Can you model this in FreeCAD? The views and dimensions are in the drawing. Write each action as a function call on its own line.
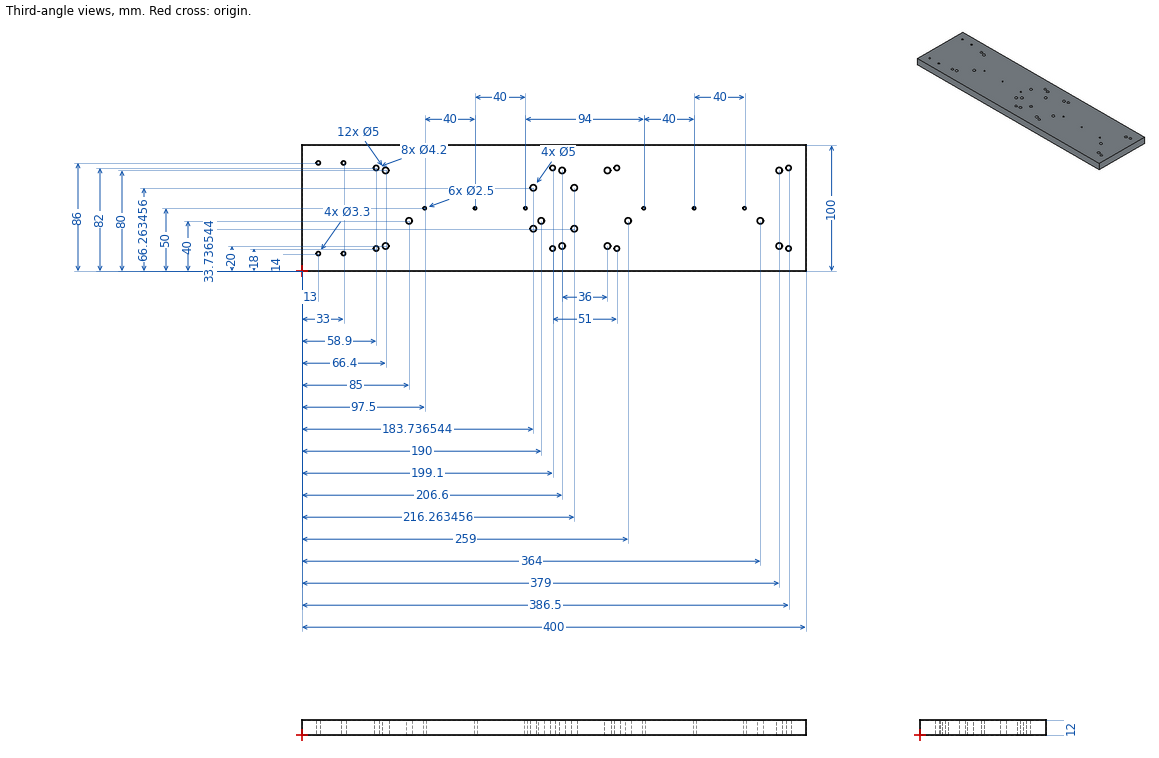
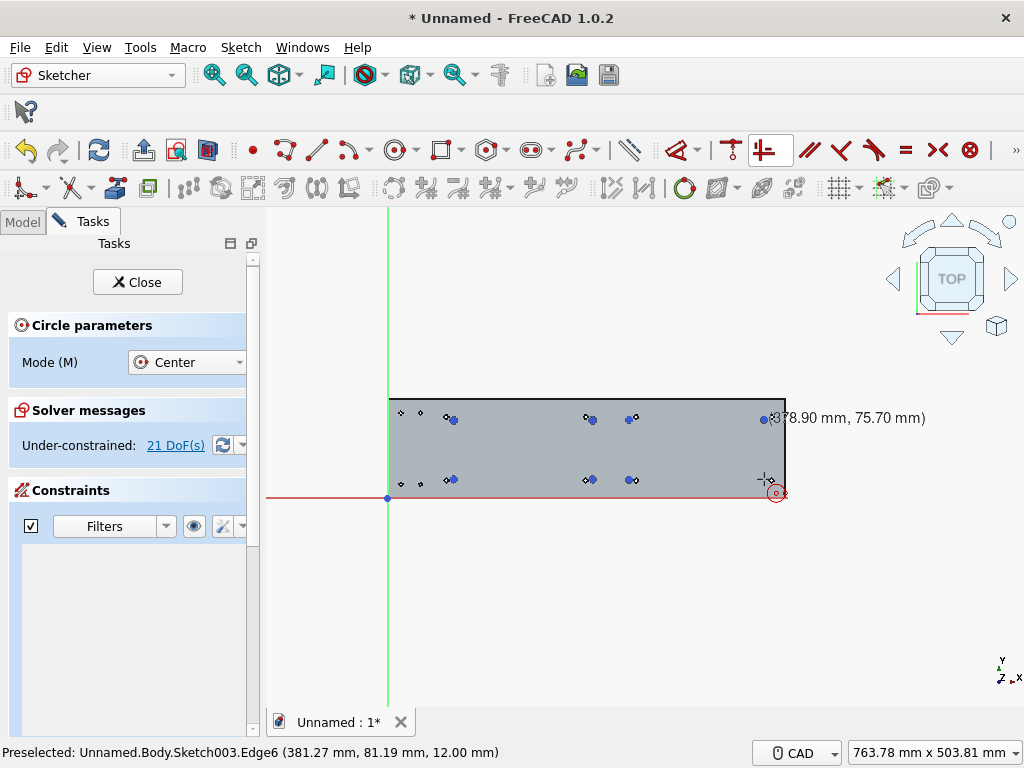
click(764, 479)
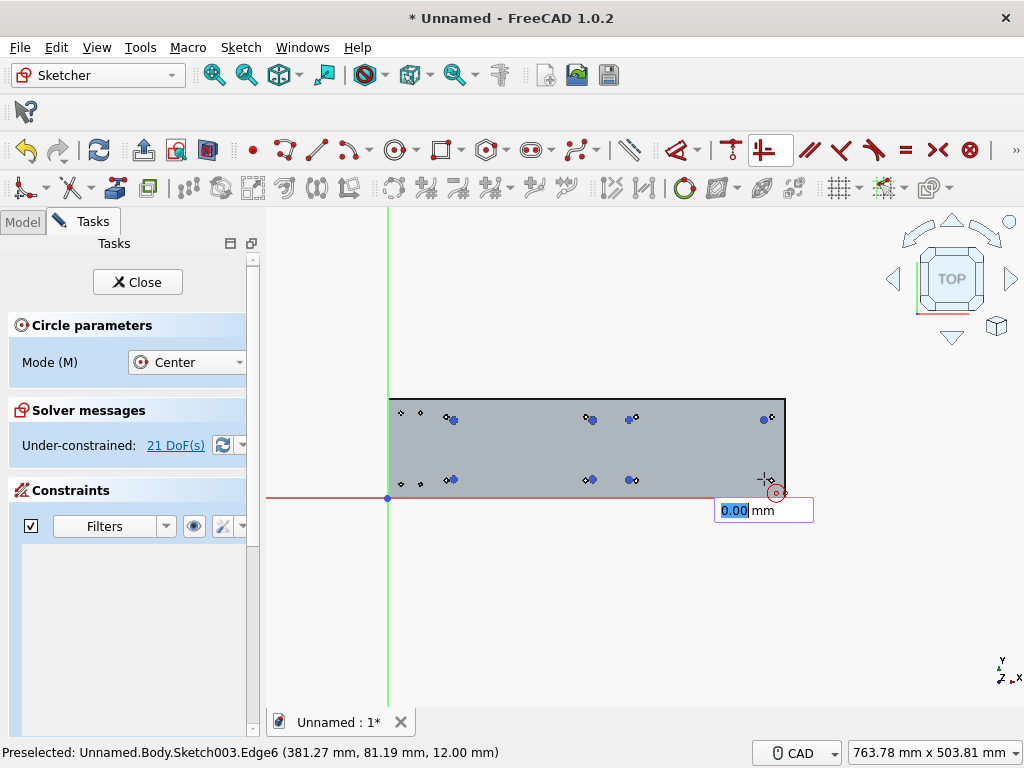
scroll(766, 477, up, 10)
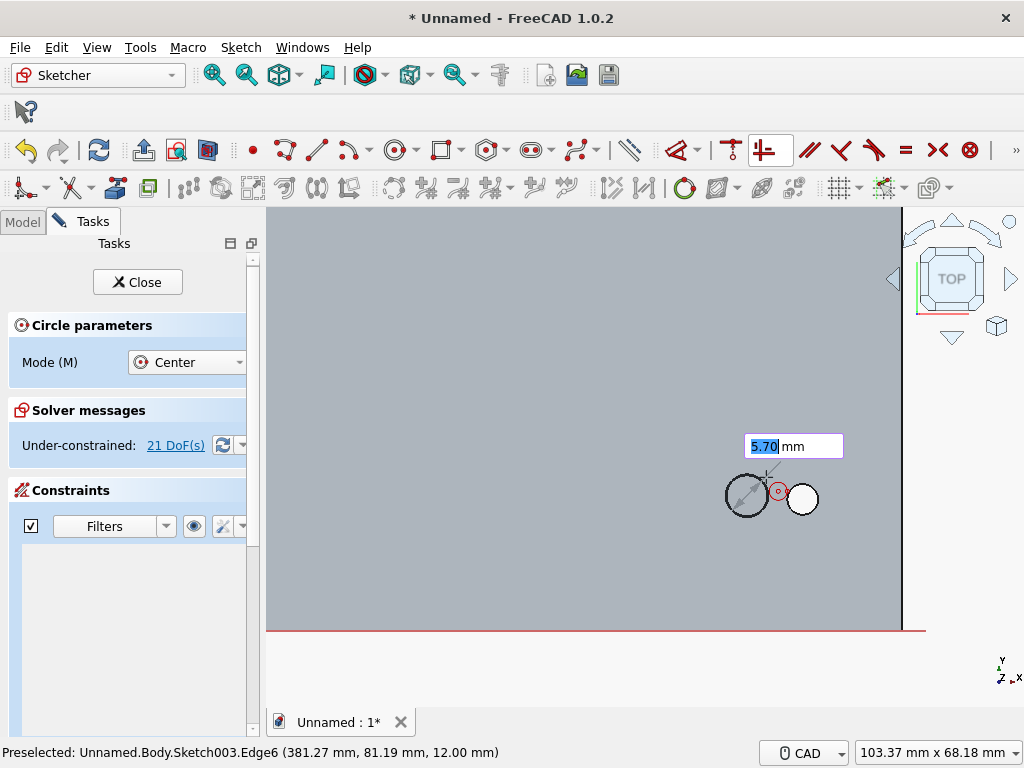
click(761, 472)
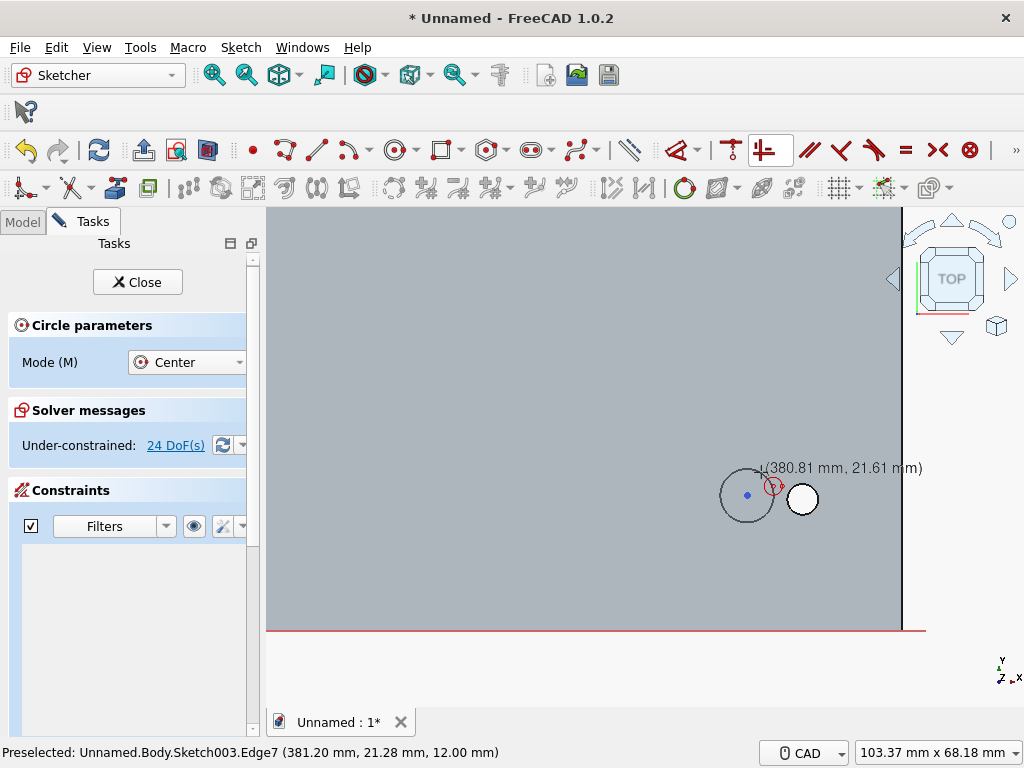
scroll(766, 477, down, 10)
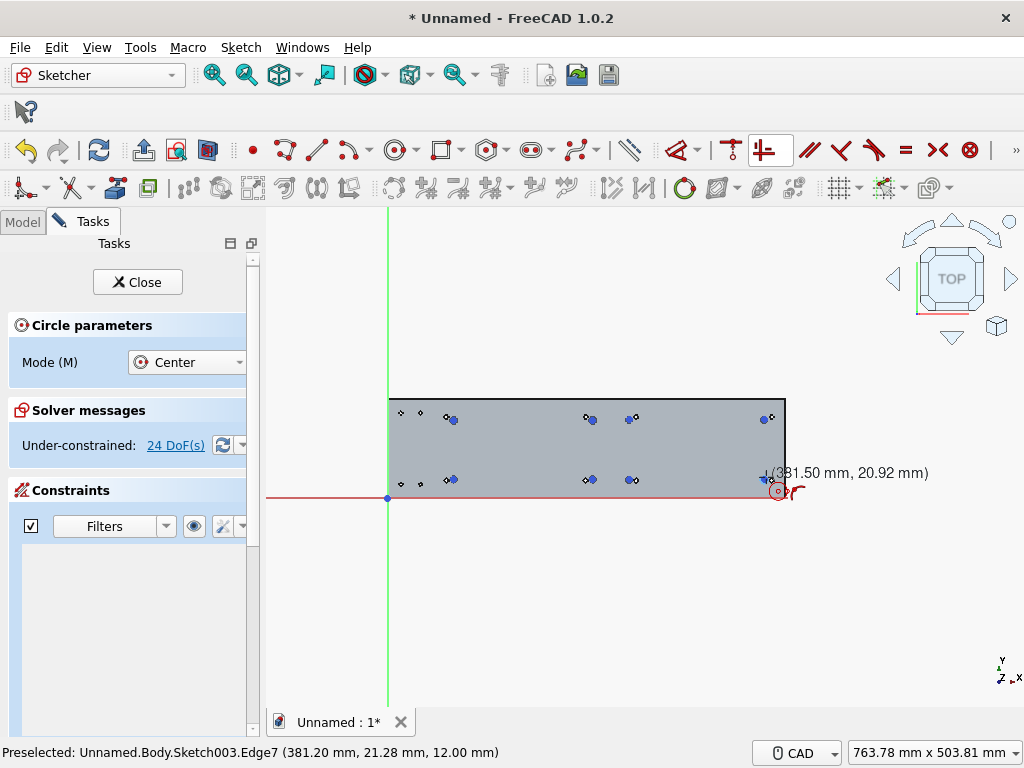
scroll(472, 459, up, 12)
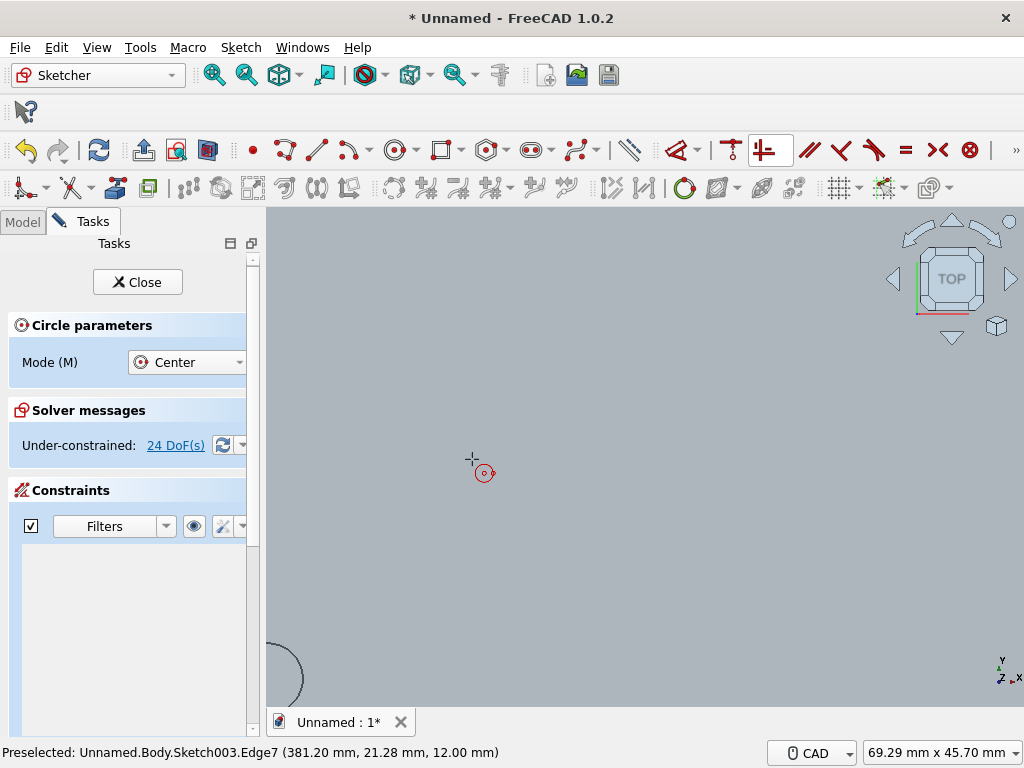
scroll(471, 459, down, 12)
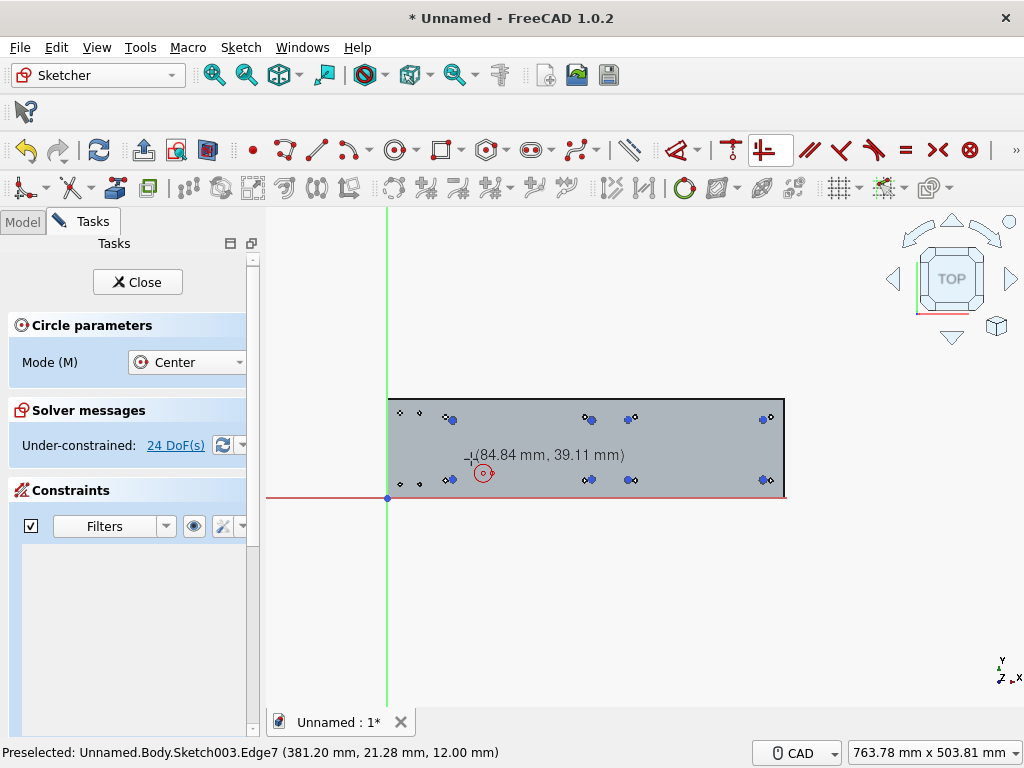
click(471, 459)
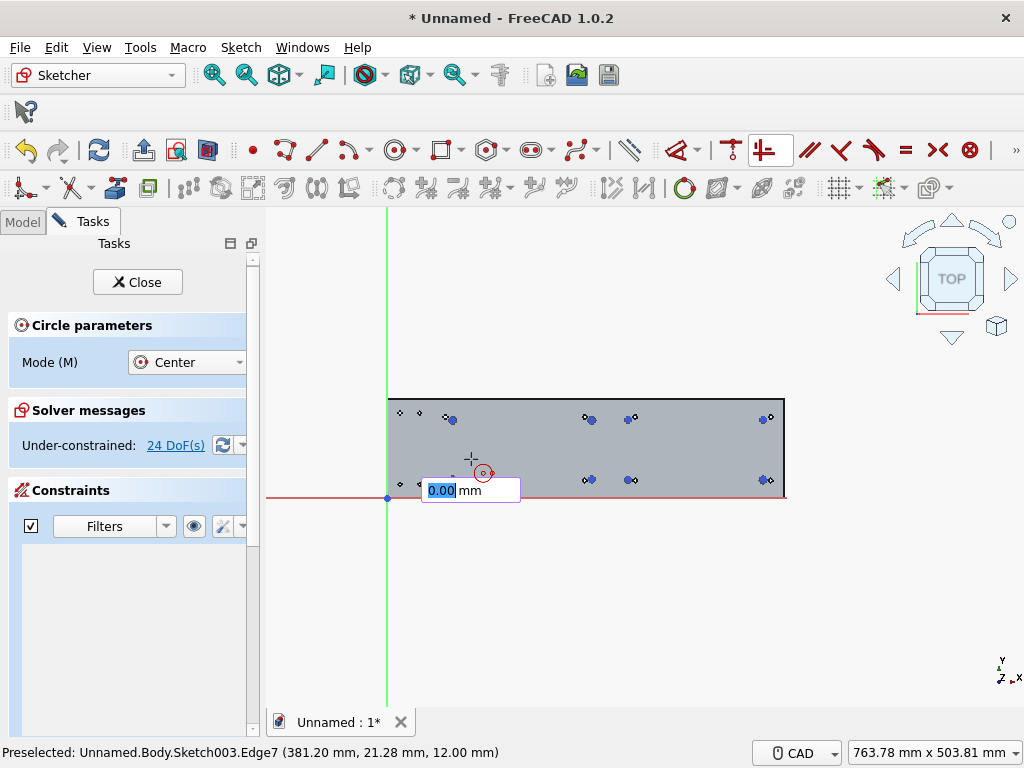
scroll(473, 457, up, 10)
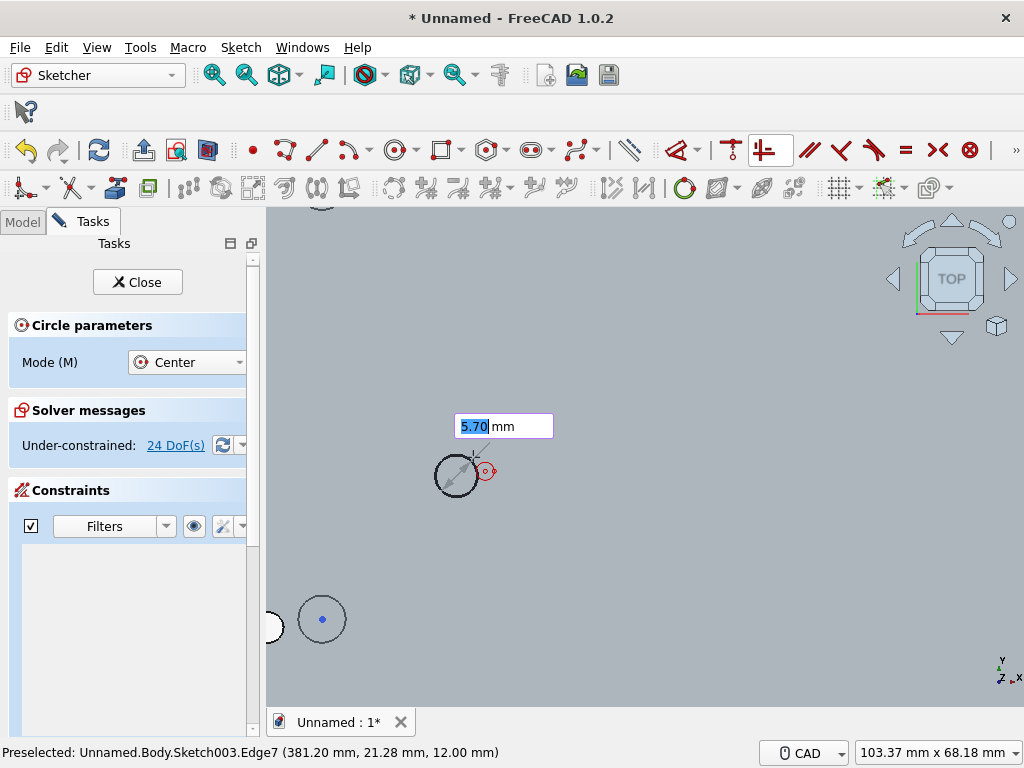
click(472, 453)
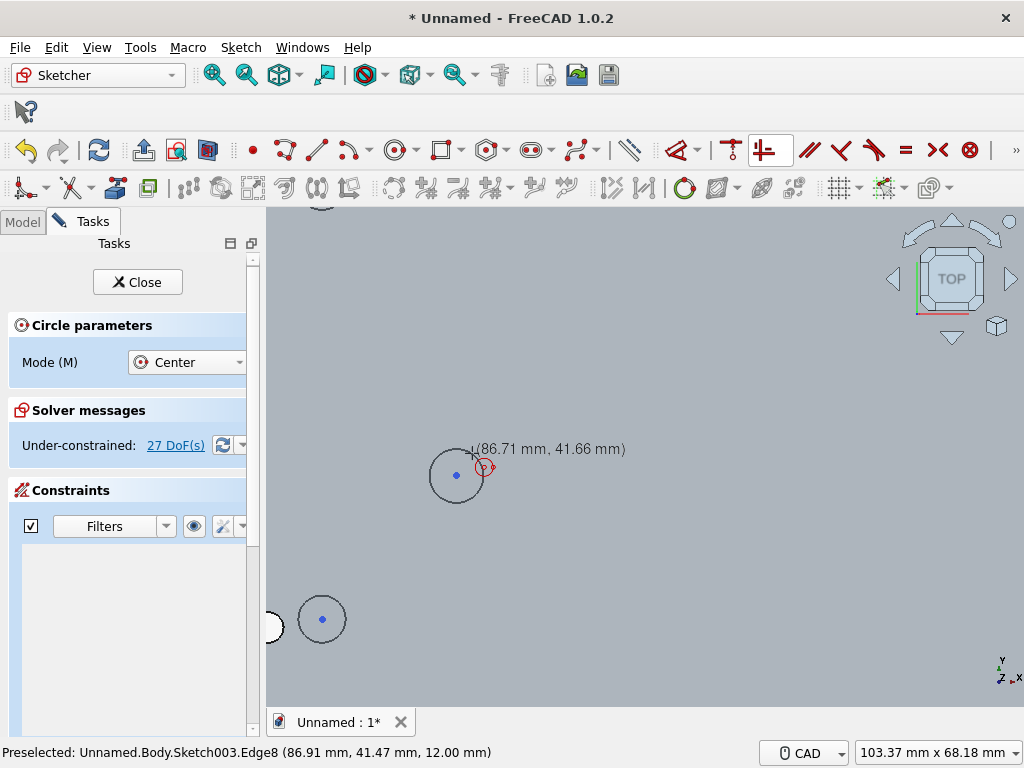
scroll(473, 457, down, 10)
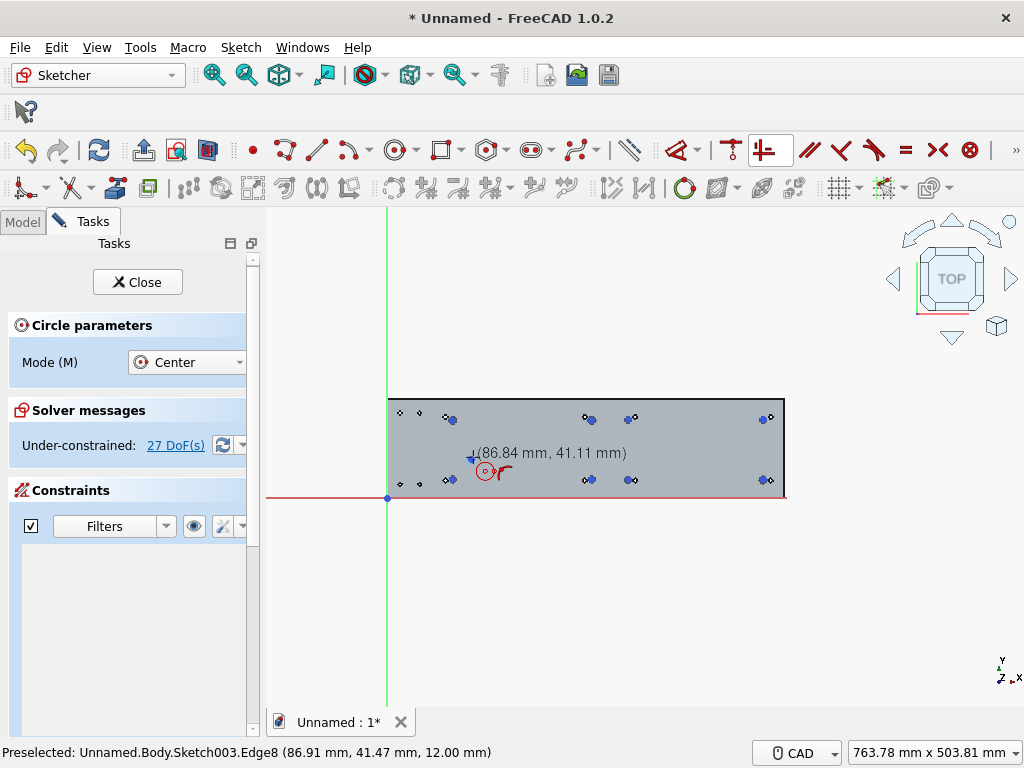
scroll(576, 459, up, 12)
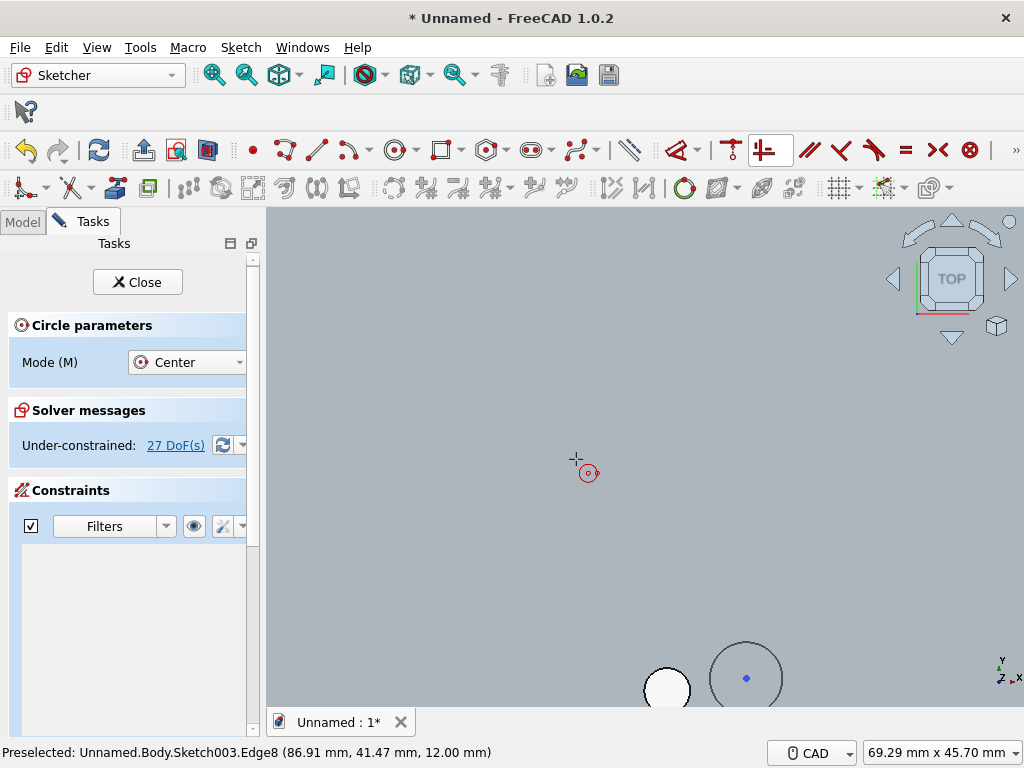
scroll(577, 459, down, 12)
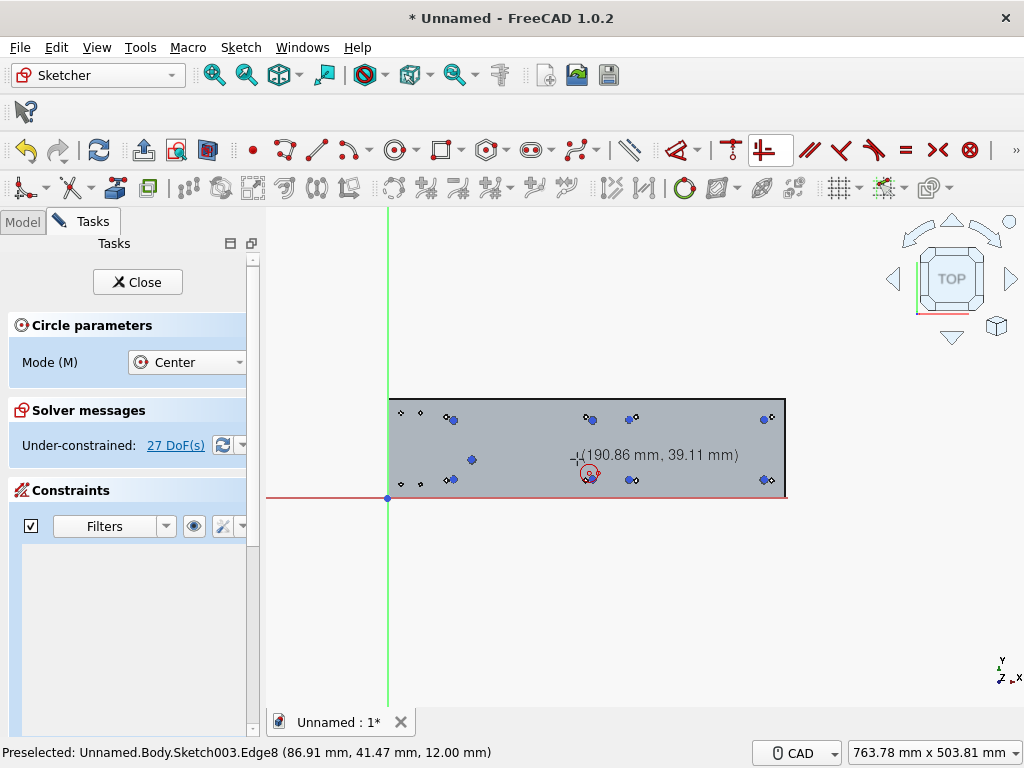
click(577, 459)